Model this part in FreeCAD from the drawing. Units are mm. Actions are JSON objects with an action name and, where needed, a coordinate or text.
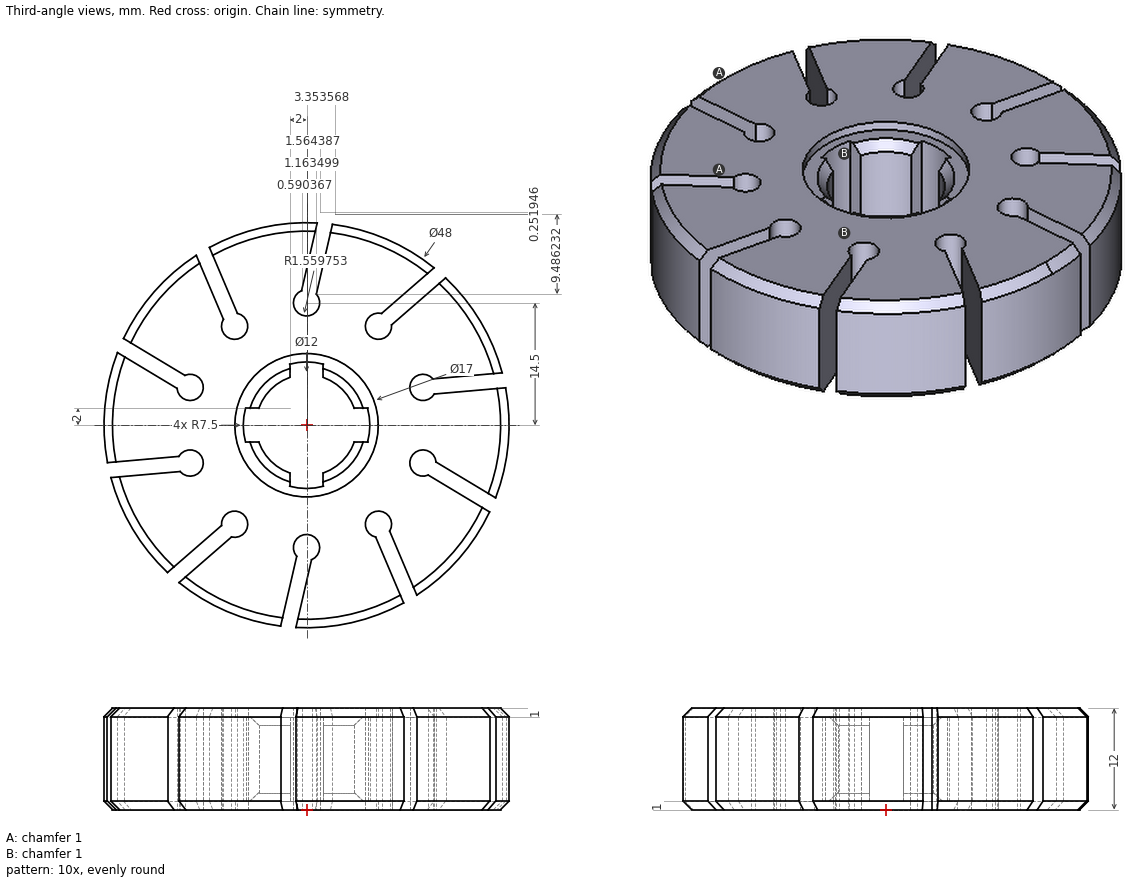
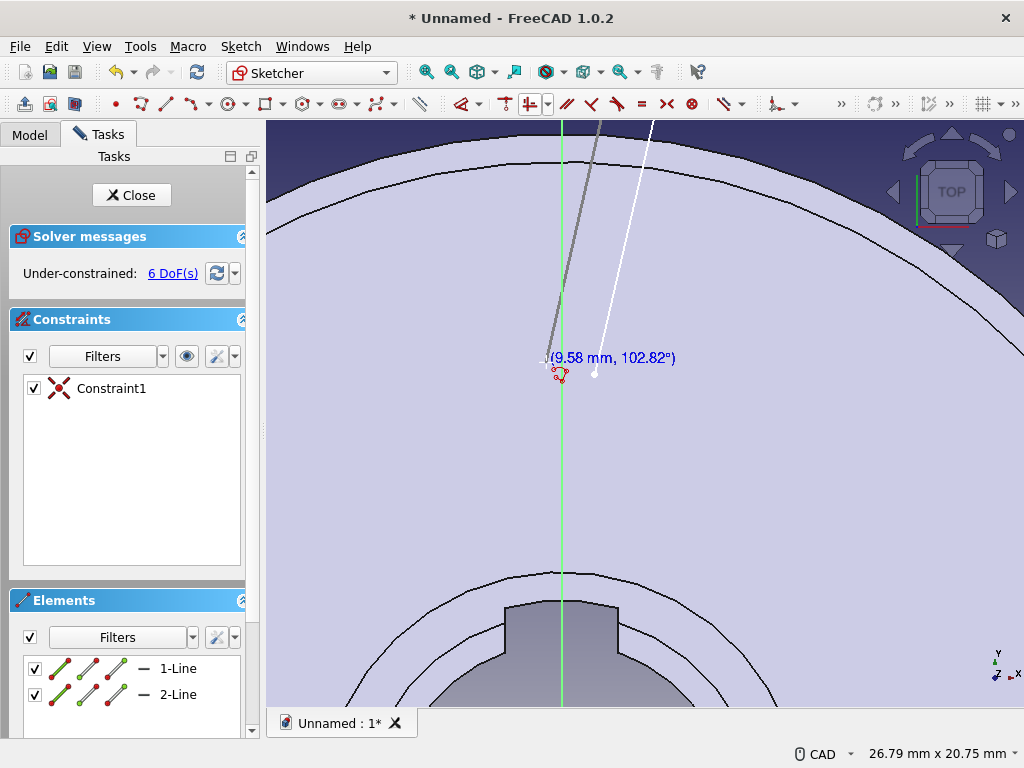
{"action": "left_click", "coordinate": [545, 362]}
{"action": "right_click", "coordinate": [545, 362]}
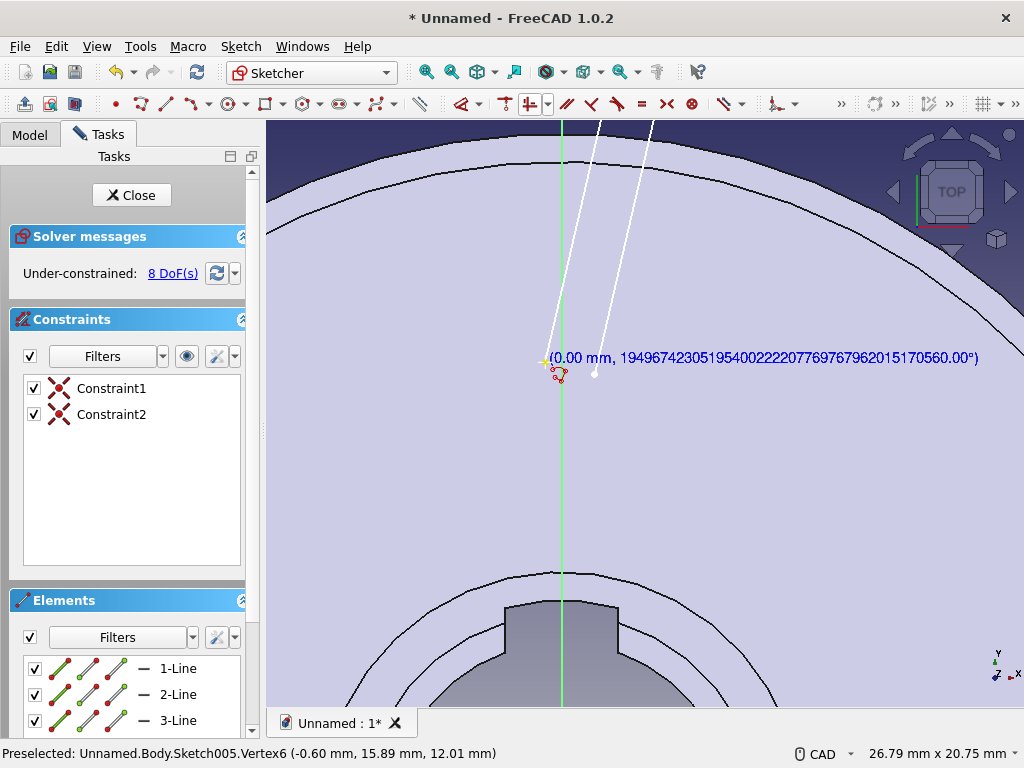
{"action": "left_click", "coordinate": [190, 104]}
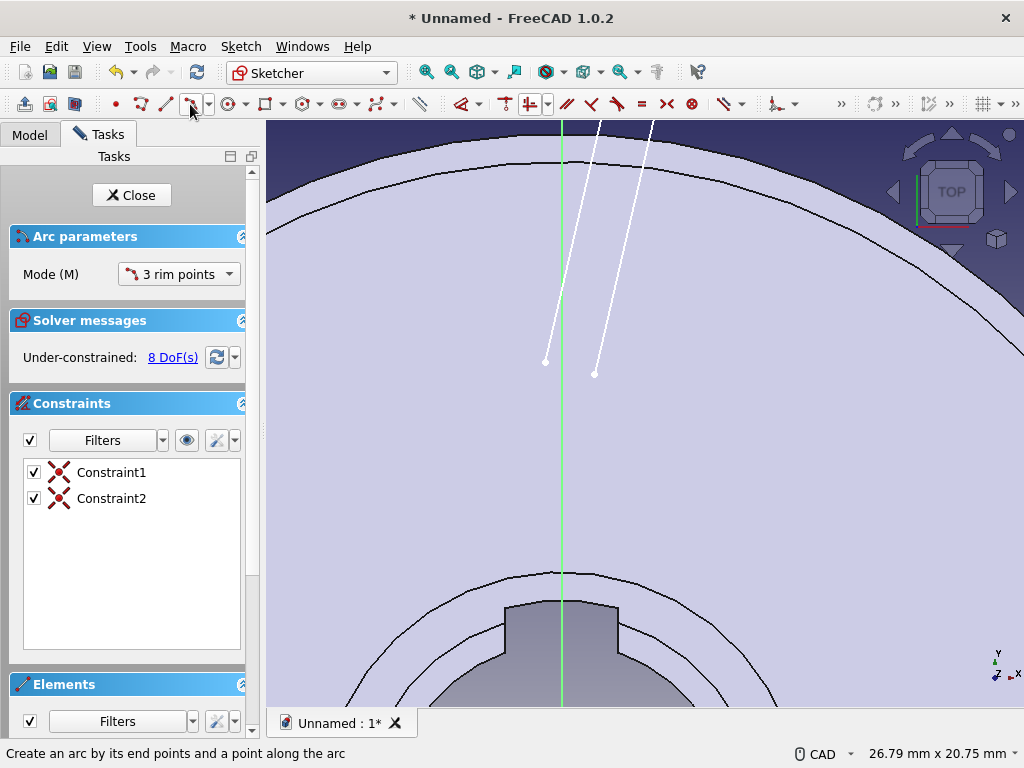
{"action": "left_click", "coordinate": [545, 363]}
{"action": "left_click", "coordinate": [595, 374]}
{"action": "left_click", "coordinate": [532, 435]}
{"action": "key", "text": "Escape"}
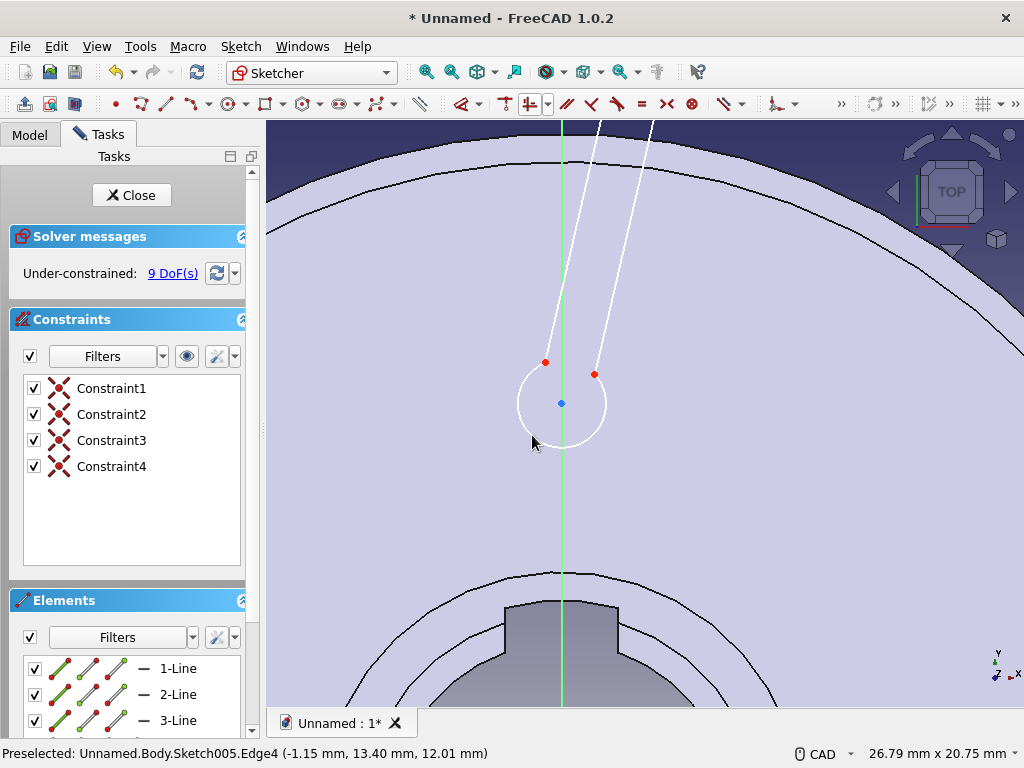
{"action": "left_click", "coordinate": [562, 404]}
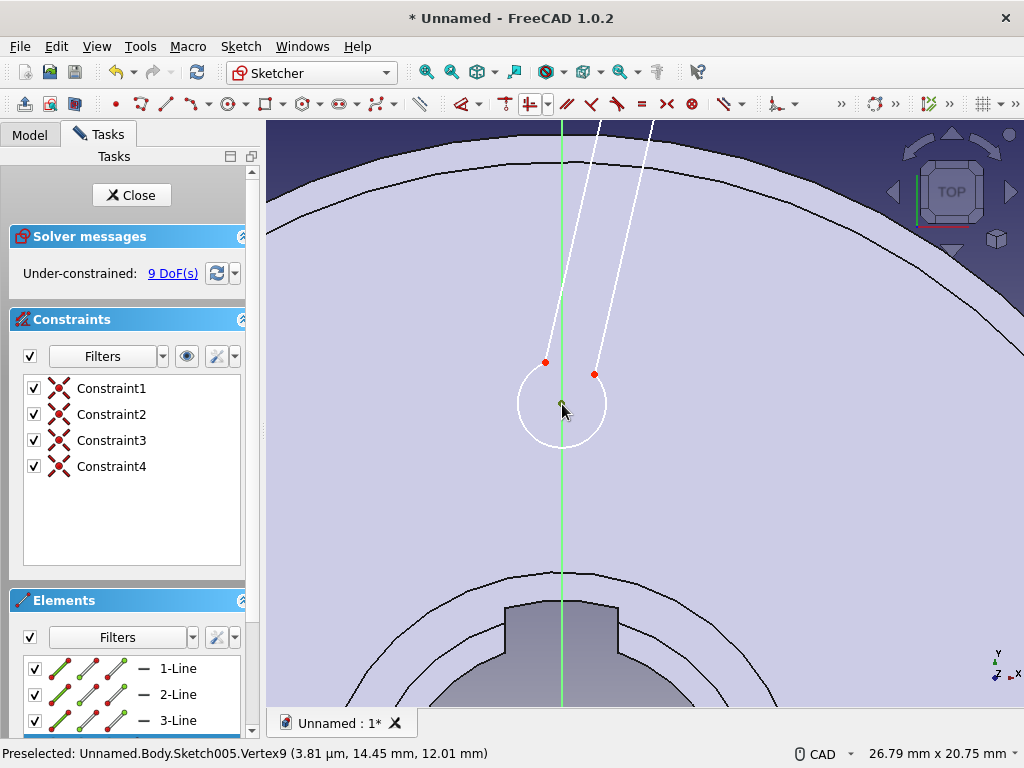
{"action": "left_click", "coordinate": [562, 641]}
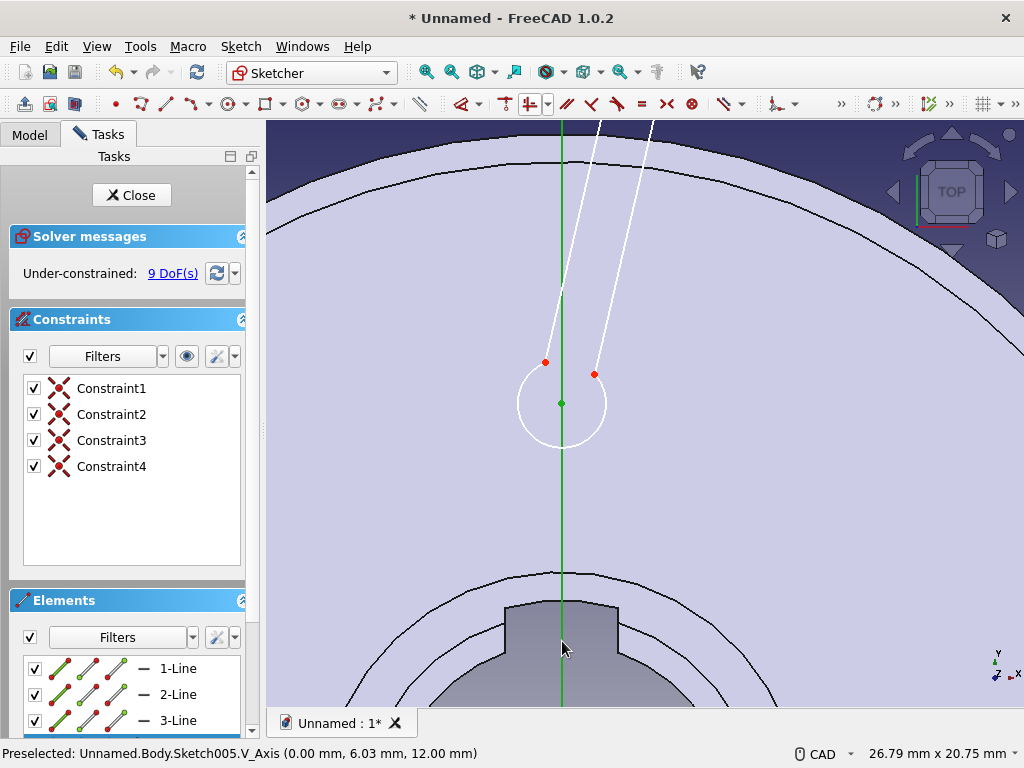
{"action": "left_click", "coordinate": [505, 104]}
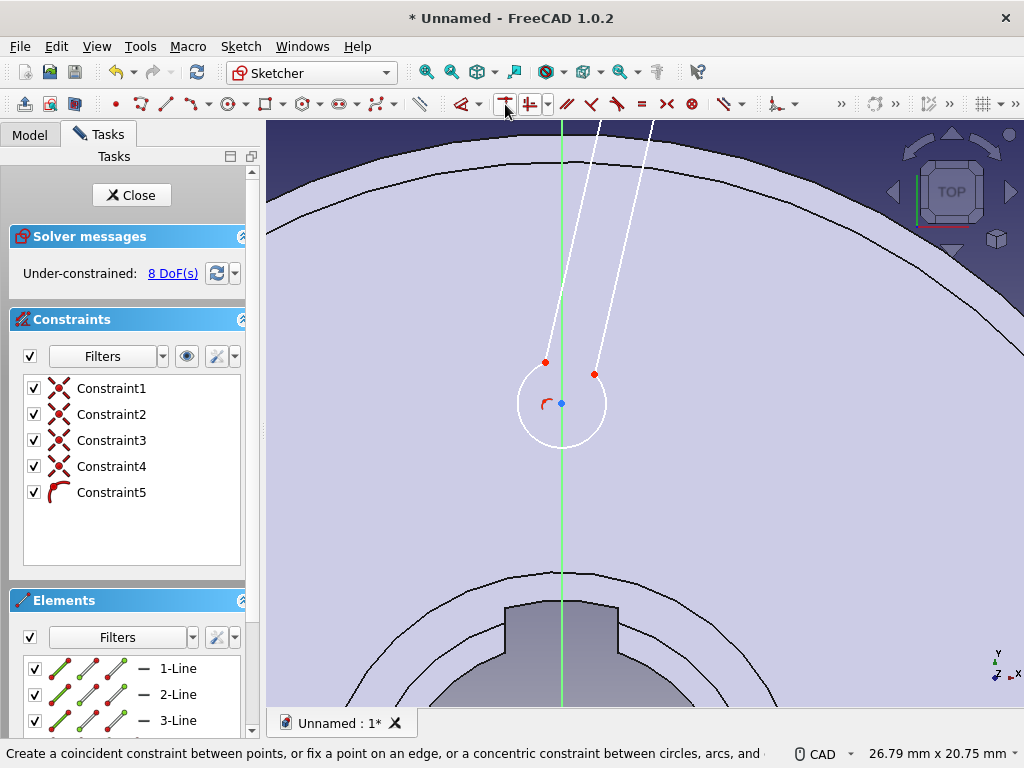
{"action": "left_click", "coordinate": [460, 104]}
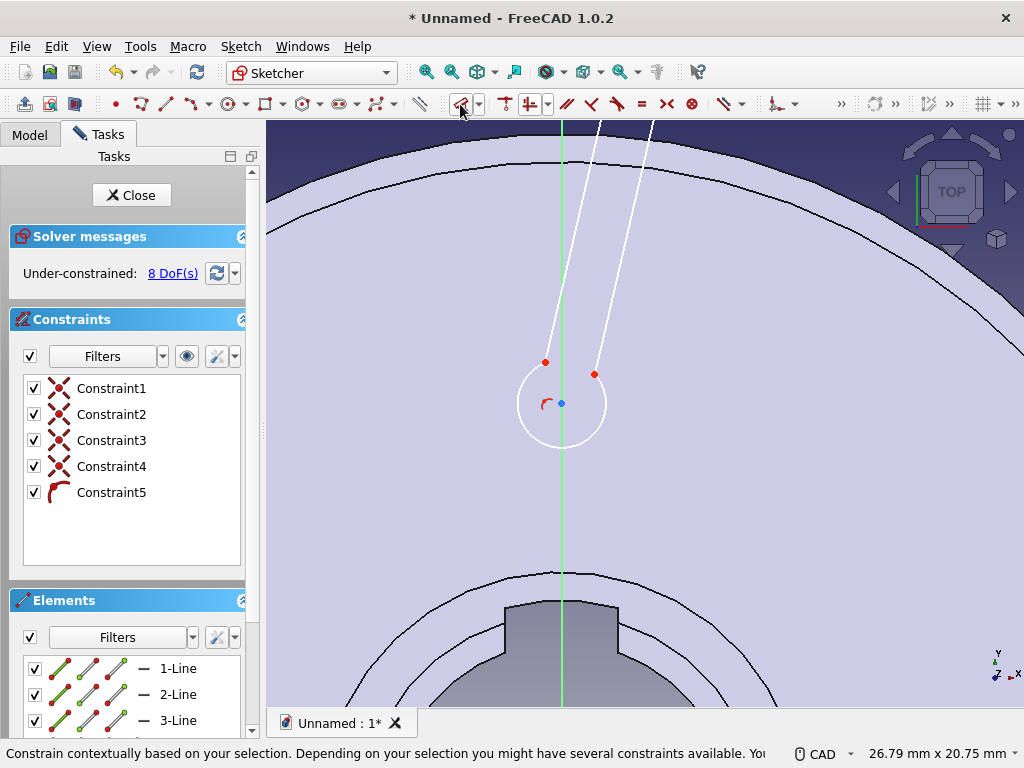
{"action": "left_click", "coordinate": [520, 418]}
{"action": "left_click", "coordinate": [490, 428]}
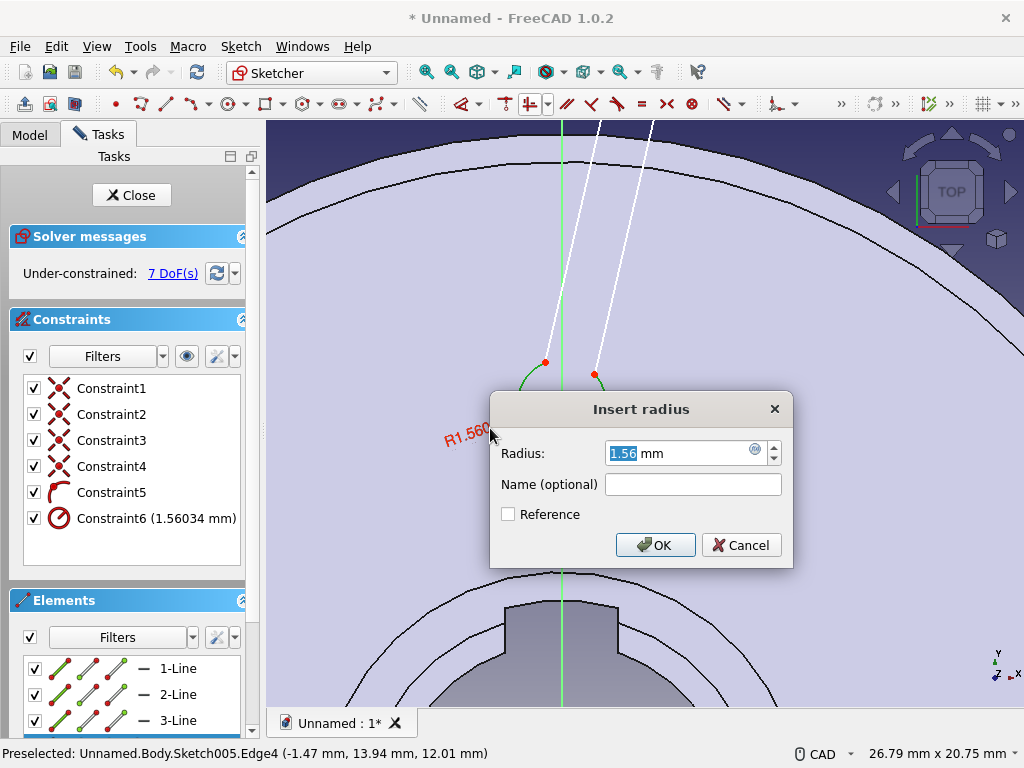
{"action": "type", "text": "1.559753"}
{"action": "key", "text": "Return"}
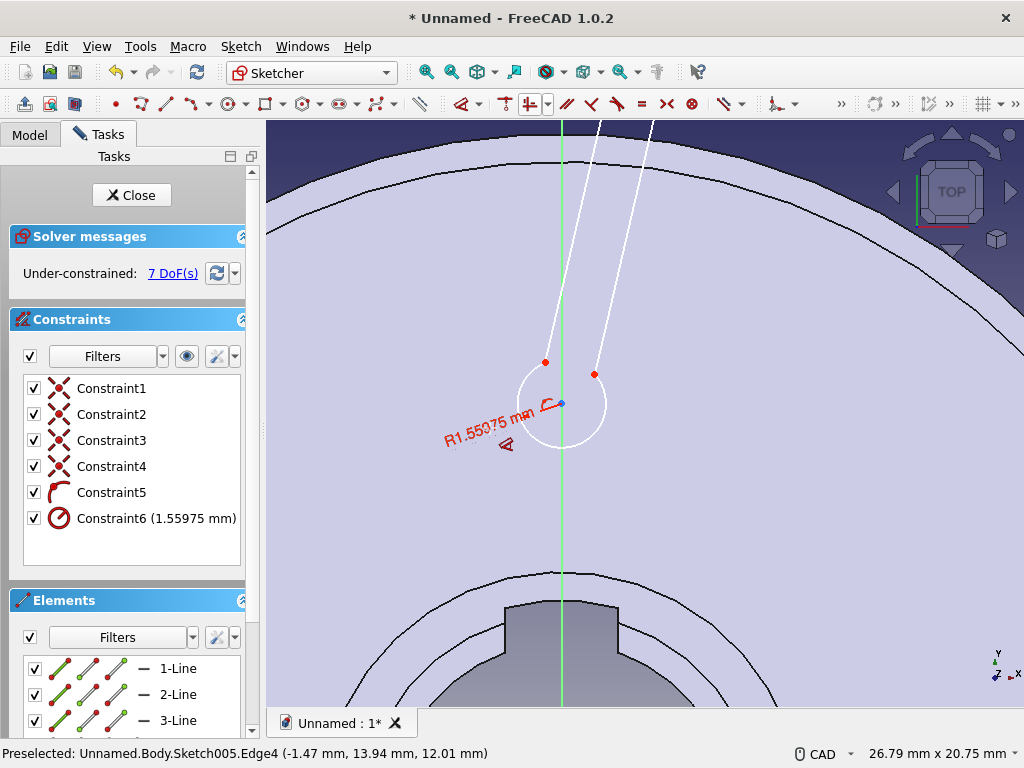
{"action": "left_click", "coordinate": [562, 404]}
{"action": "left_click", "coordinate": [528, 541]}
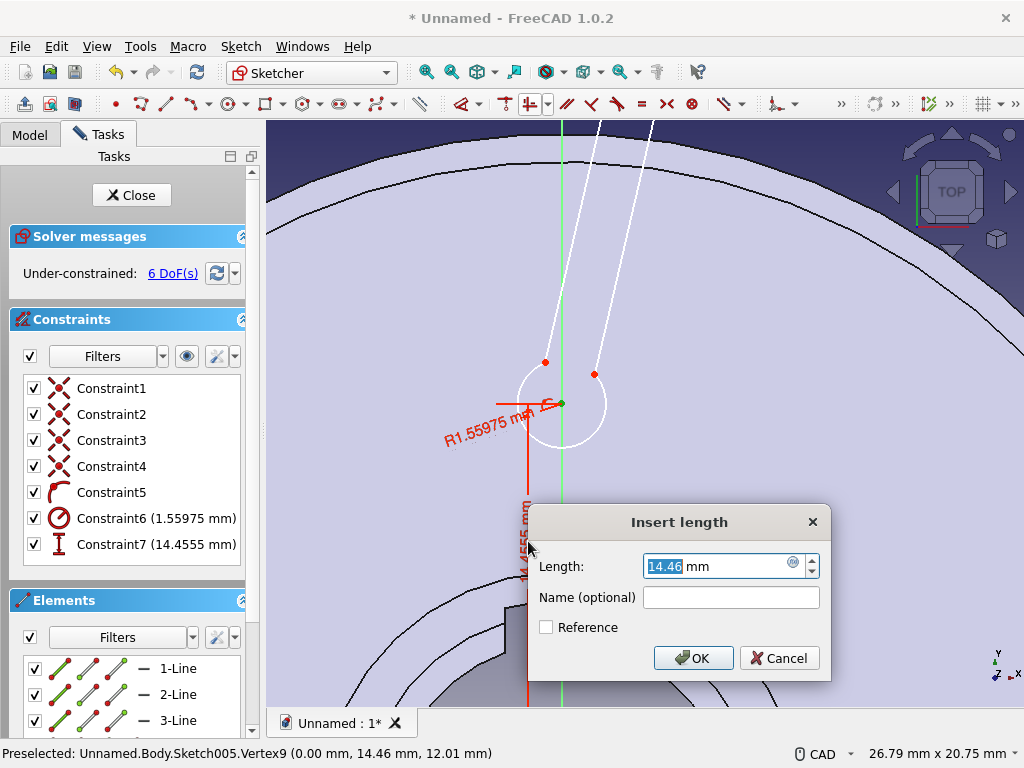
{"action": "type", "text": "14.5"}
{"action": "key", "text": "Return"}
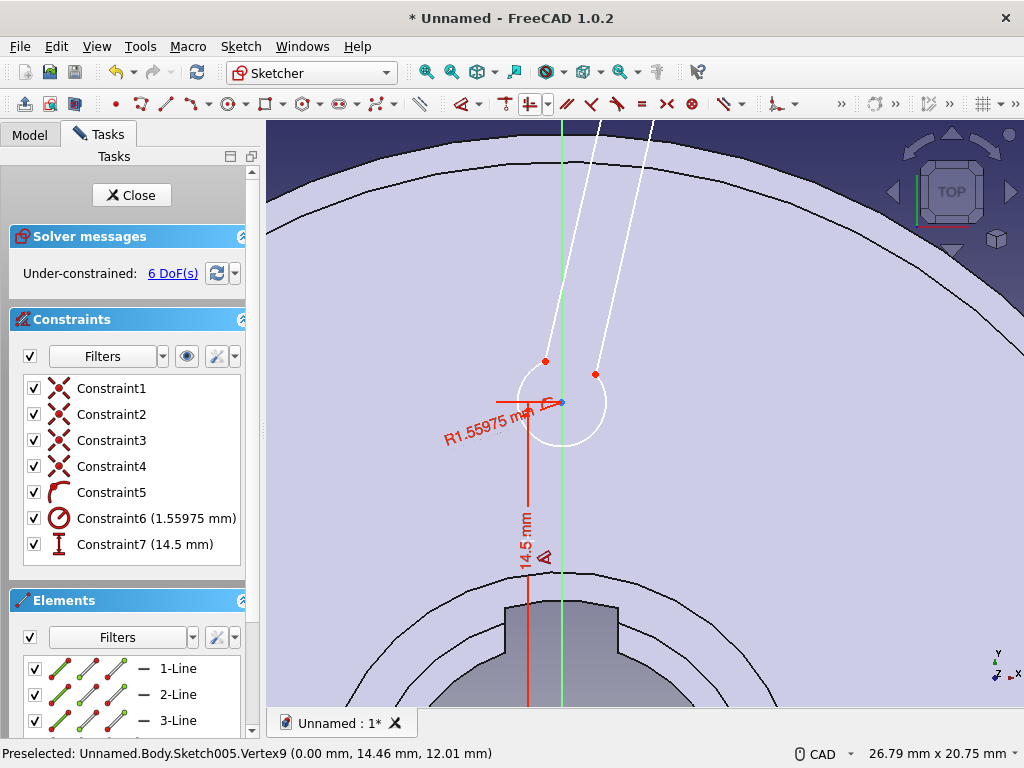
{"action": "left_click", "coordinate": [596, 374]}
{"action": "left_click", "coordinate": [579, 340]}